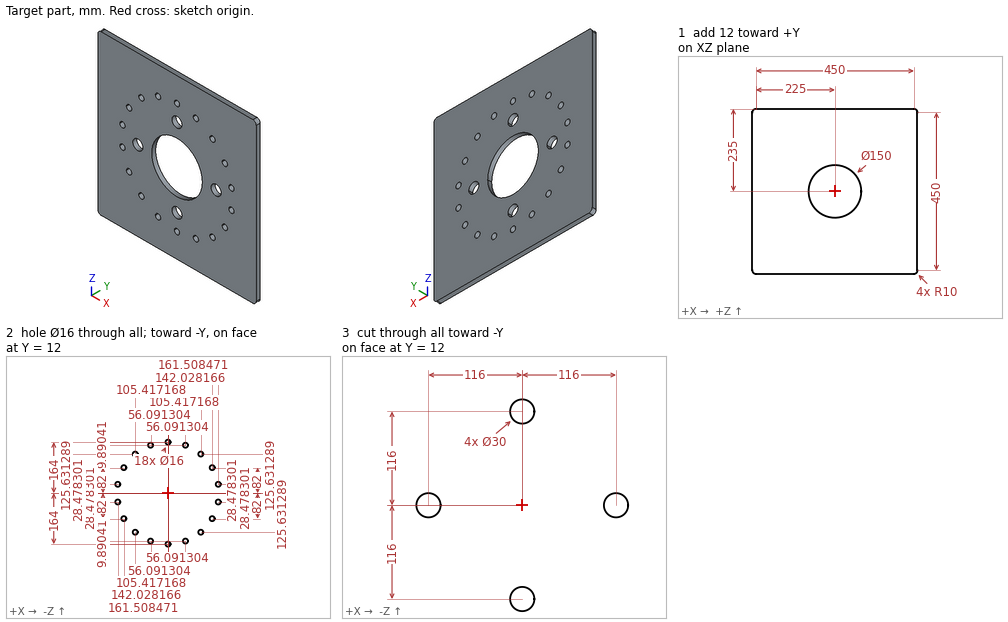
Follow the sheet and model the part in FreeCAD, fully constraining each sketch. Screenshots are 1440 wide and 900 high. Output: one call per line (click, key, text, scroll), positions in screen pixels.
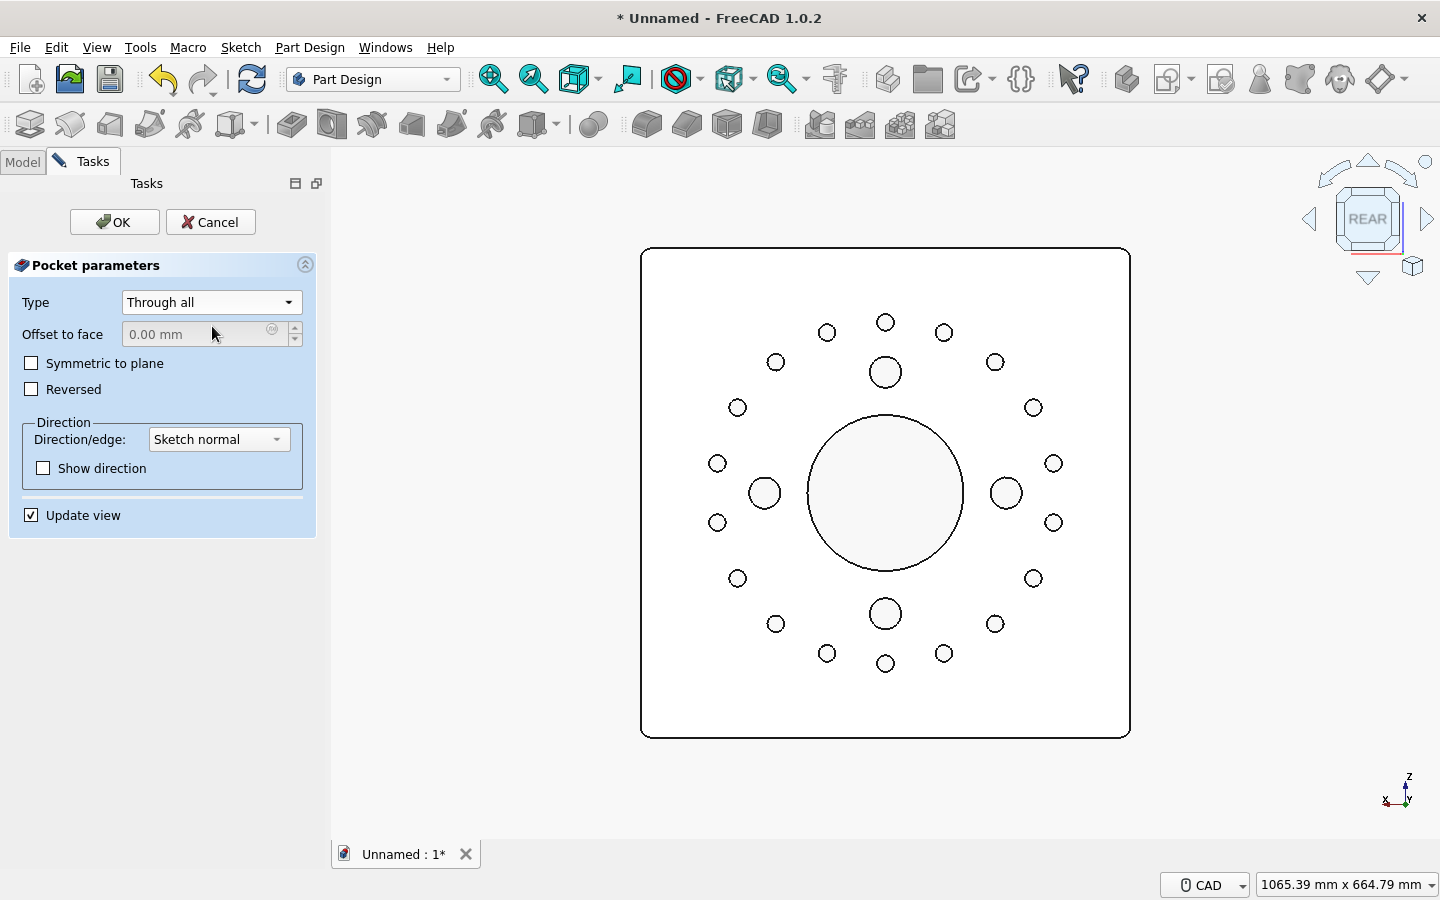
click(115, 222)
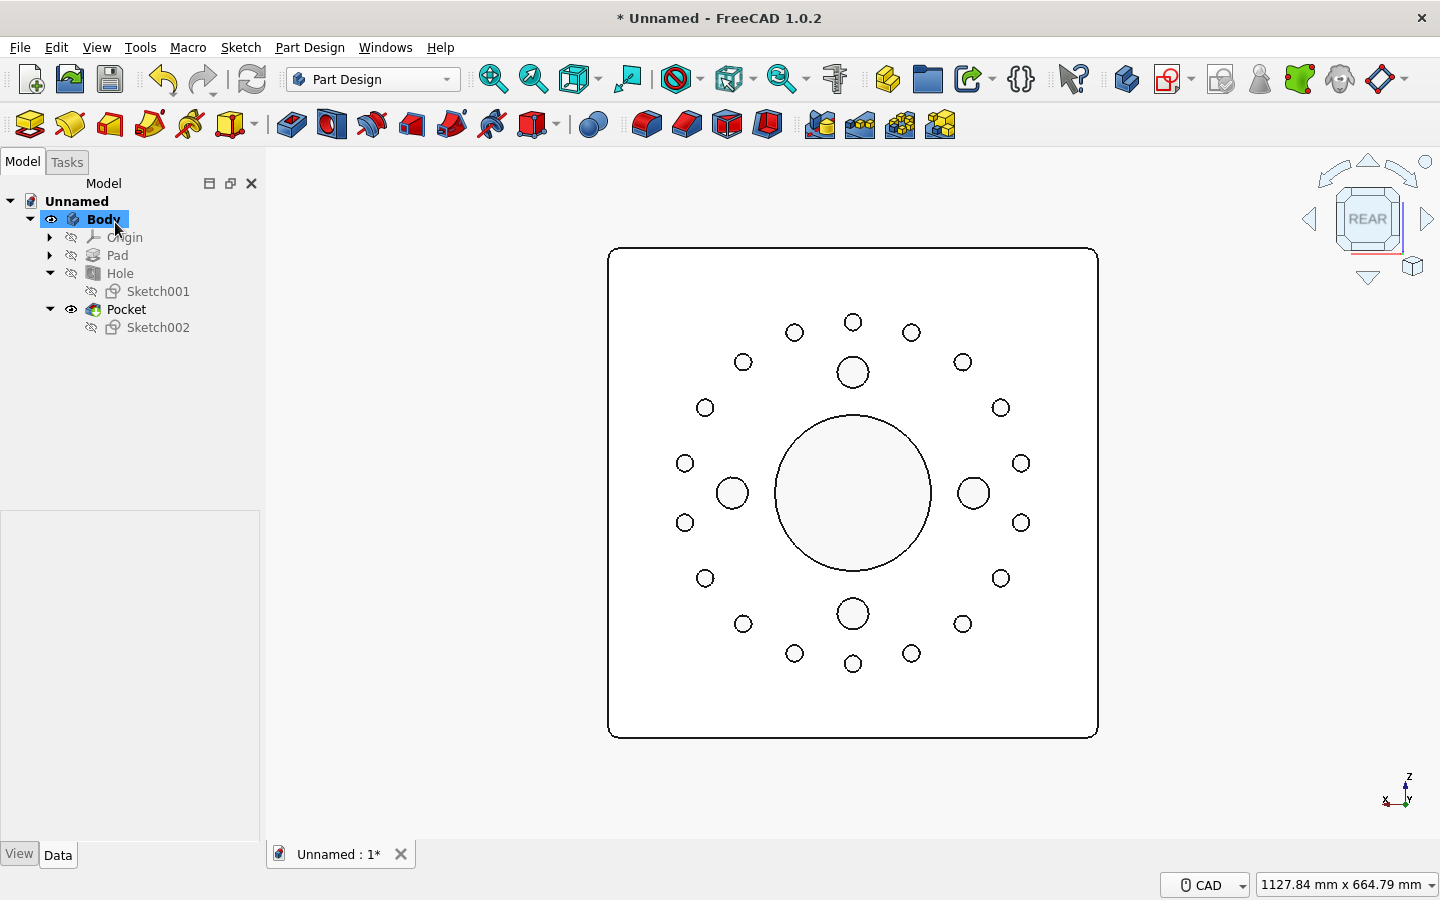
key(0)